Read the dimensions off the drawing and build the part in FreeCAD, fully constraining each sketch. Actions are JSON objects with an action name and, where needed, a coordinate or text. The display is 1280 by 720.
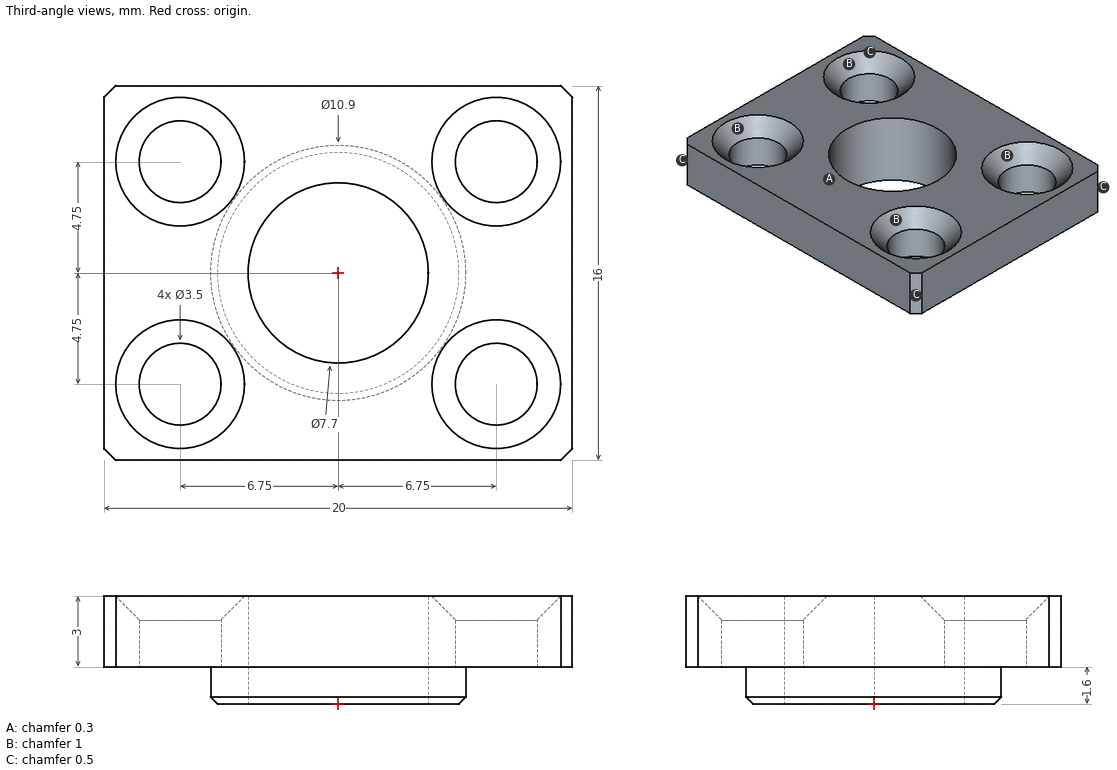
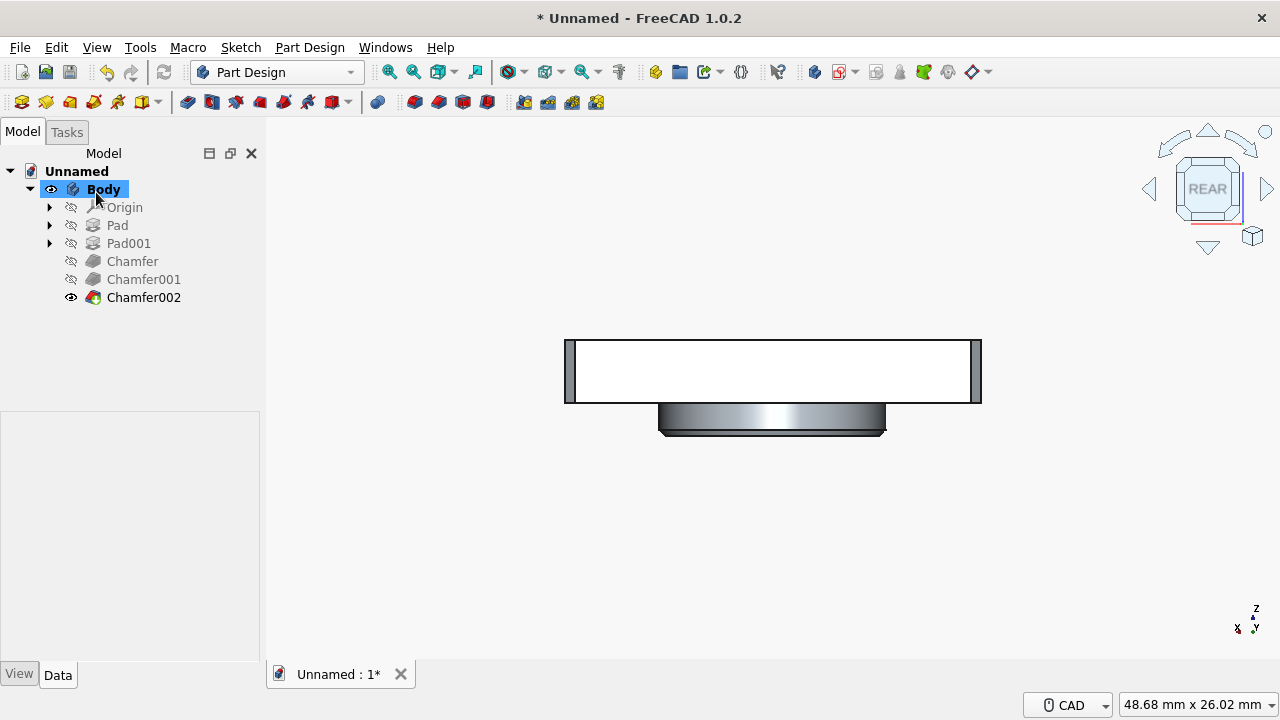
{"action": "key", "text": "0"}